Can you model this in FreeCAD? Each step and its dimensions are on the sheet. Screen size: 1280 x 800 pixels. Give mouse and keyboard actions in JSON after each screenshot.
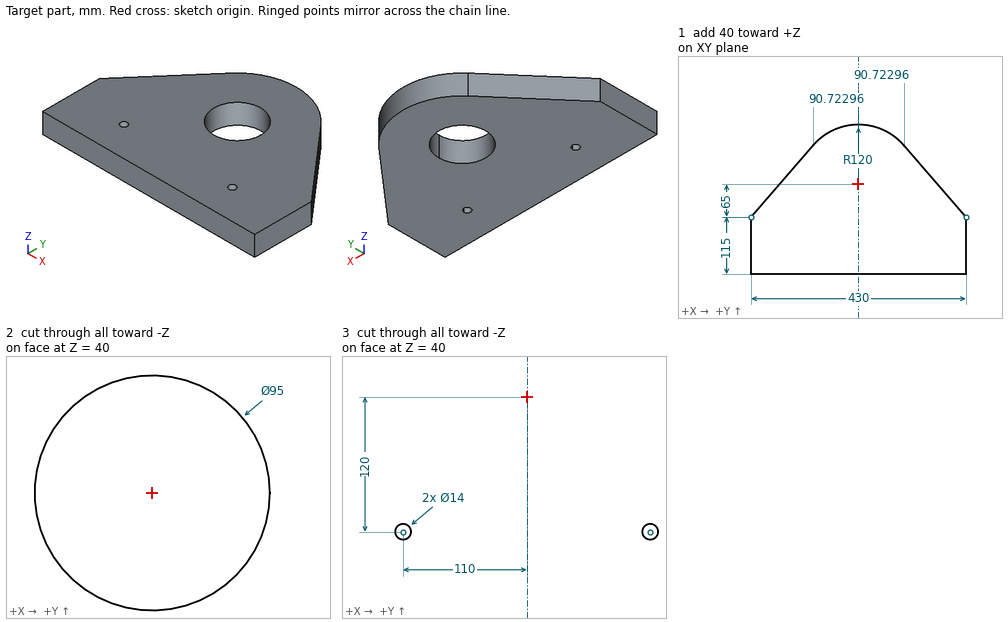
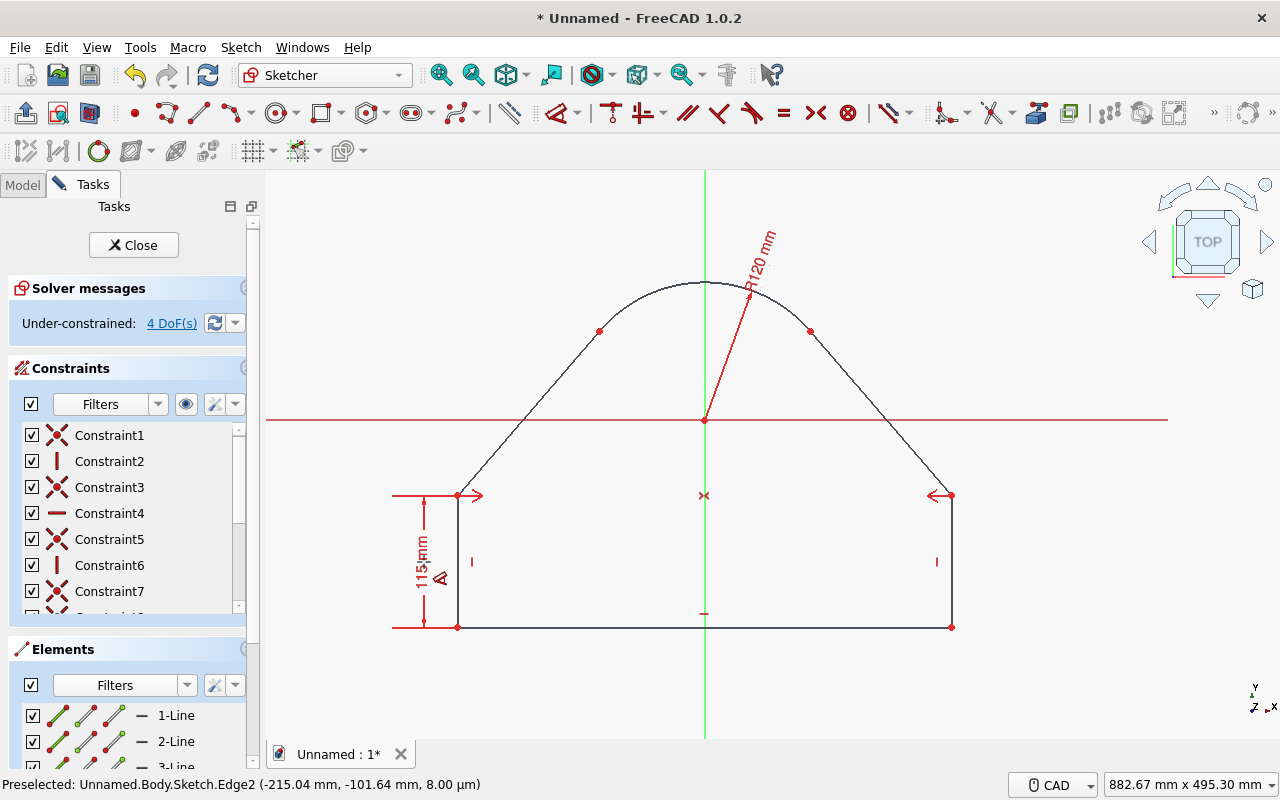
{"action": "left_click", "coordinate": [606, 628]}
{"action": "left_click", "coordinate": [591, 662]}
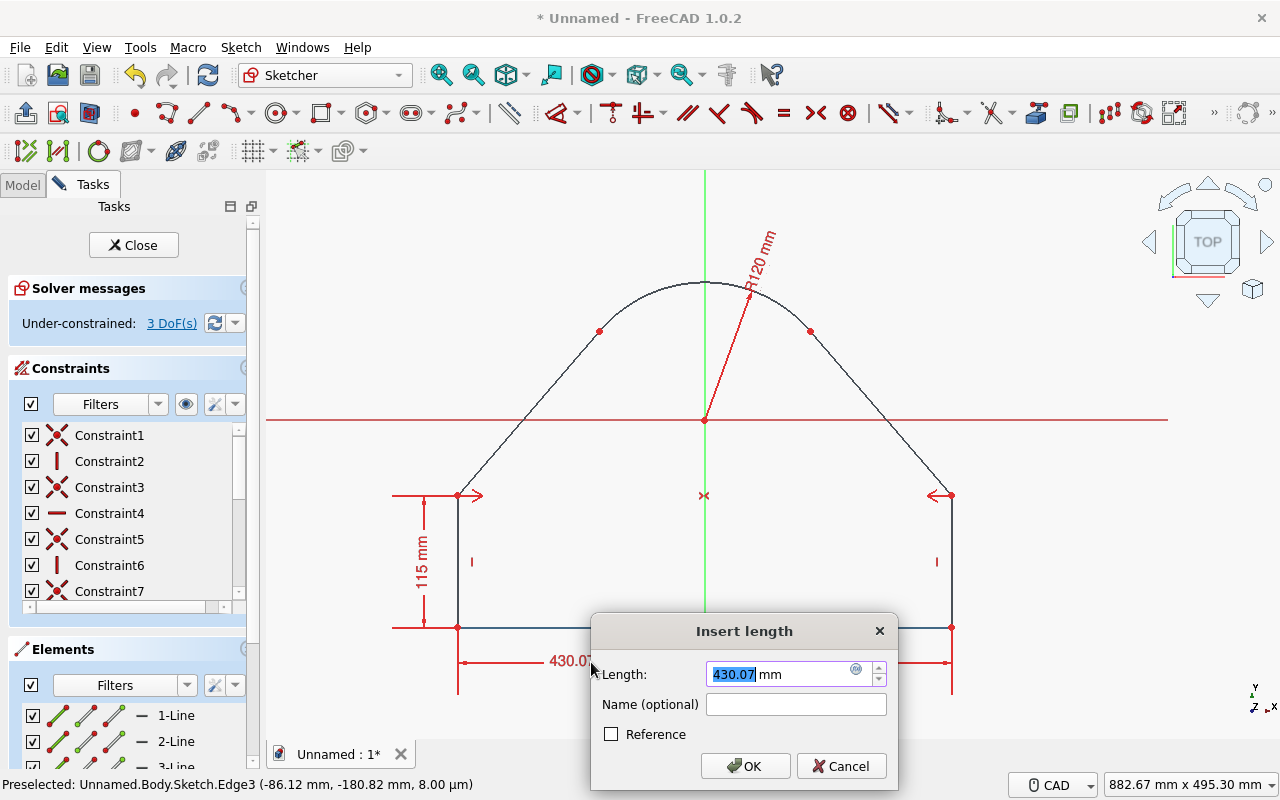
{"action": "type", "text": "430"}
{"action": "key", "text": "Return"}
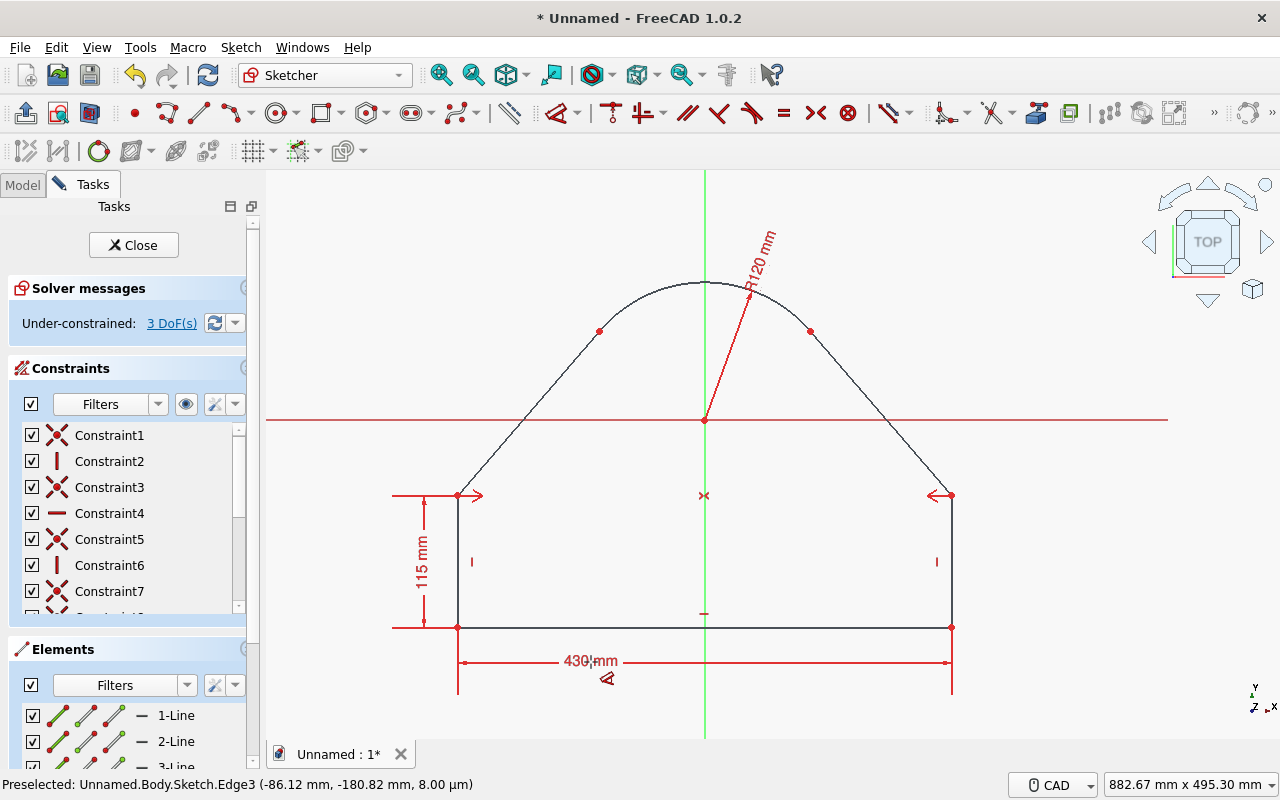
{"action": "left_click", "coordinate": [458, 496]}
{"action": "left_click", "coordinate": [424, 458]}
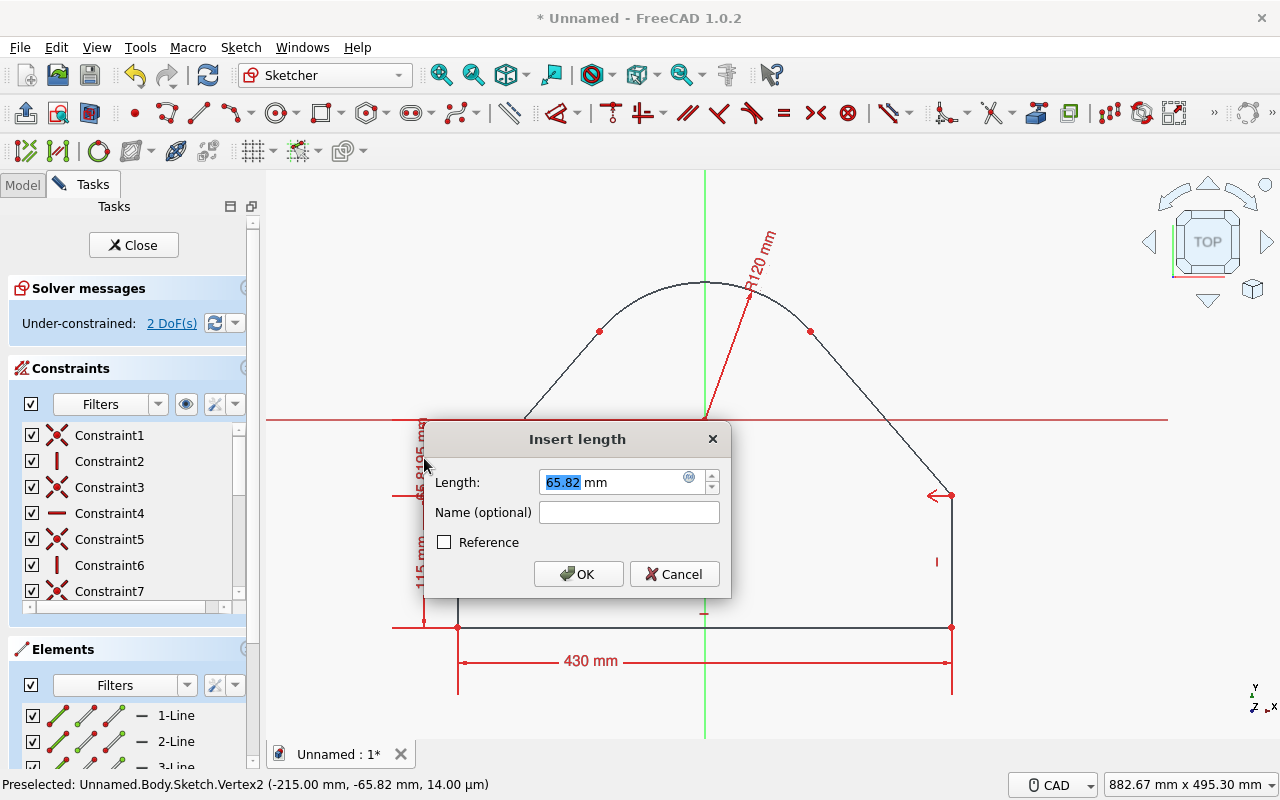
{"action": "type", "text": "65"}
{"action": "key", "text": "Return"}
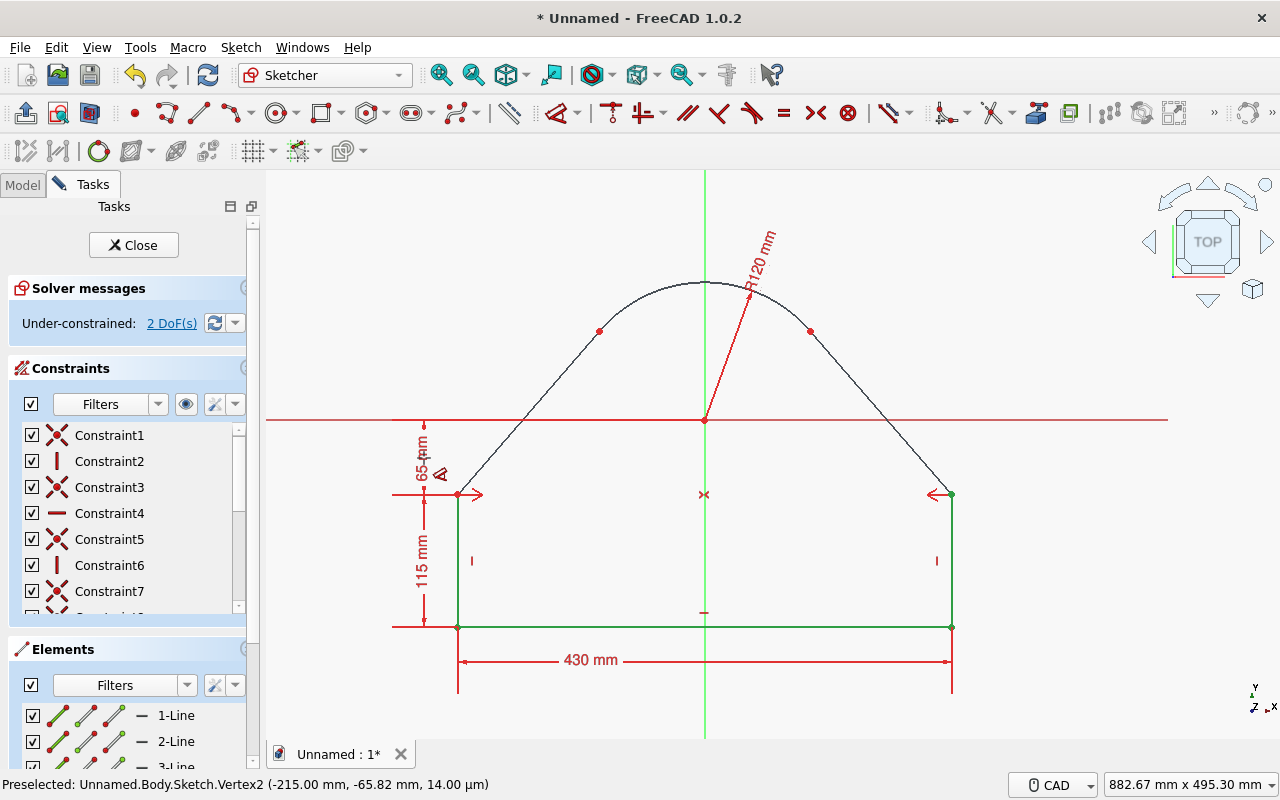
{"action": "left_click", "coordinate": [600, 331]}
{"action": "left_click", "coordinate": [615, 297]}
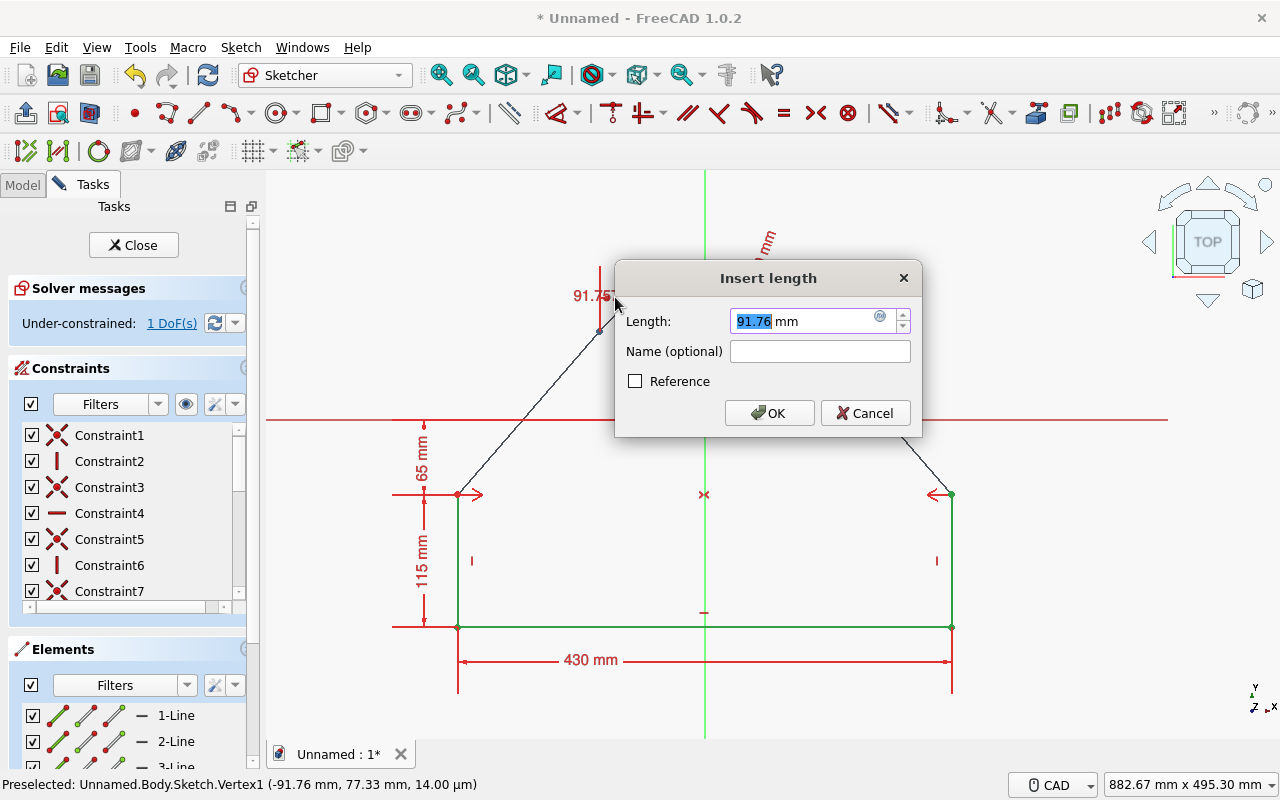
{"action": "type", "text": "90.72296"}
{"action": "key", "text": "Return"}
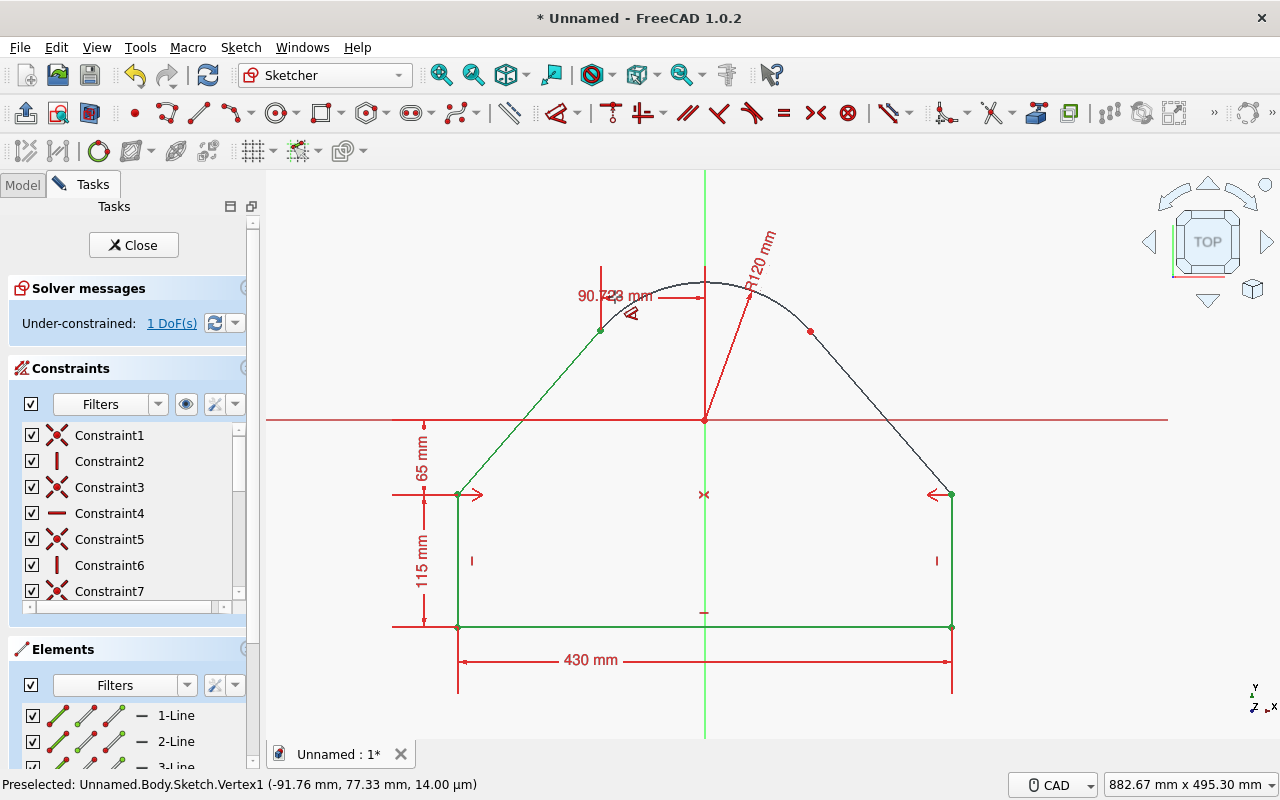
{"action": "left_click", "coordinate": [810, 331]}
{"action": "left_click", "coordinate": [721, 297]}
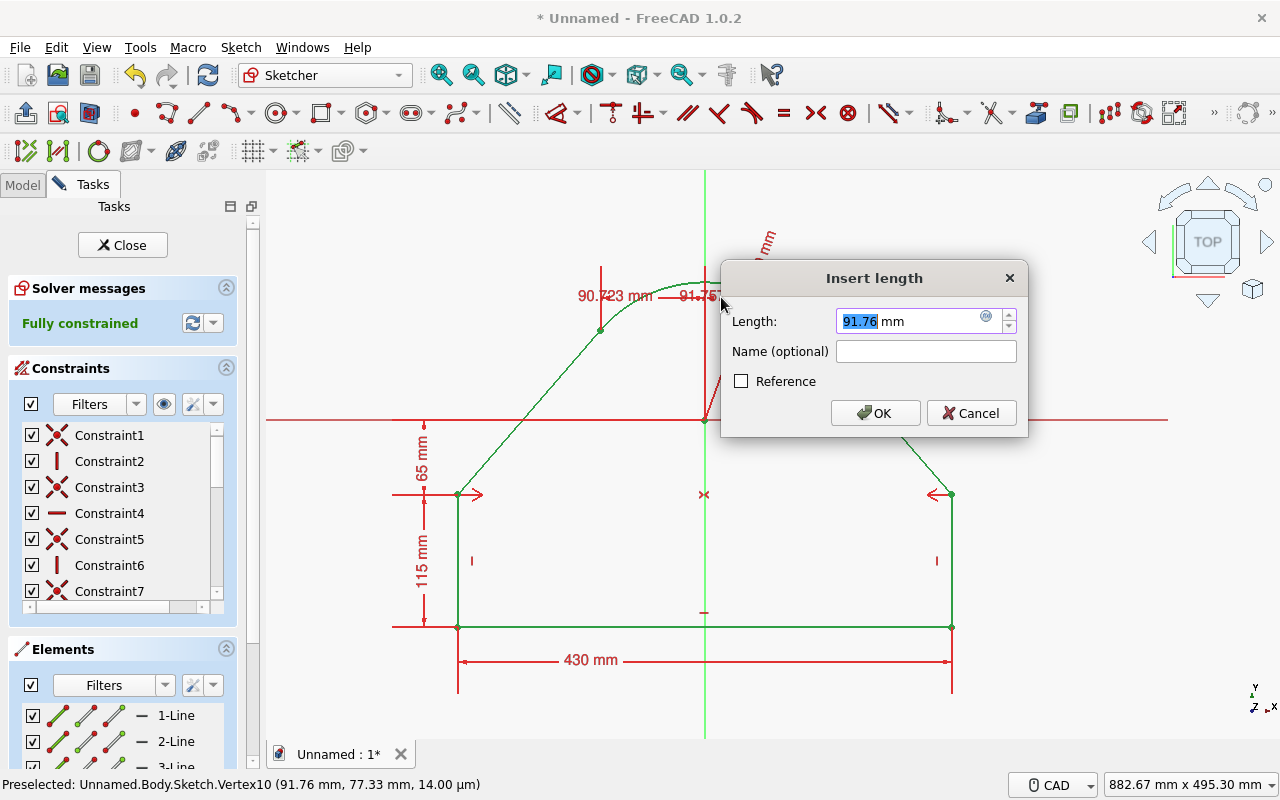
{"action": "type", "text": "90.72296"}
{"action": "key", "text": "Return"}
{"action": "key", "text": "Escape"}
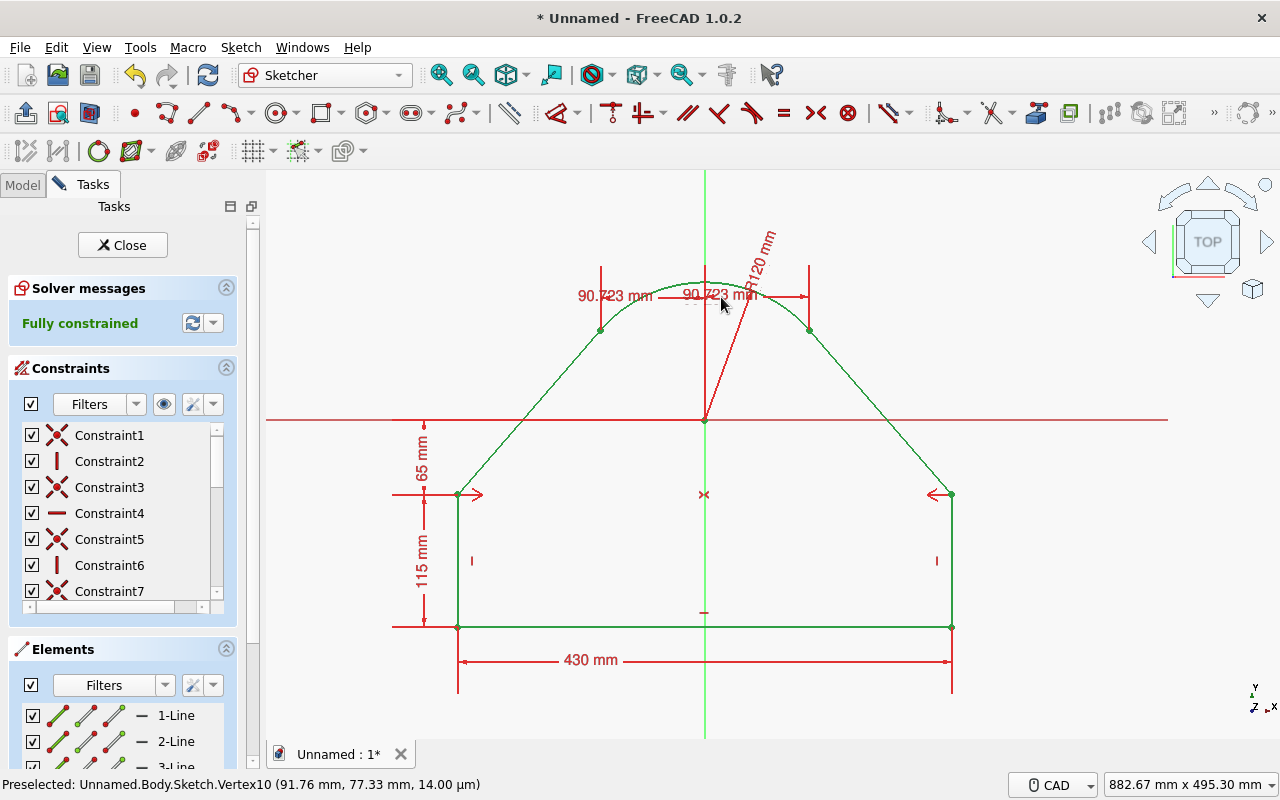
{"action": "left_click", "coordinate": [123, 245]}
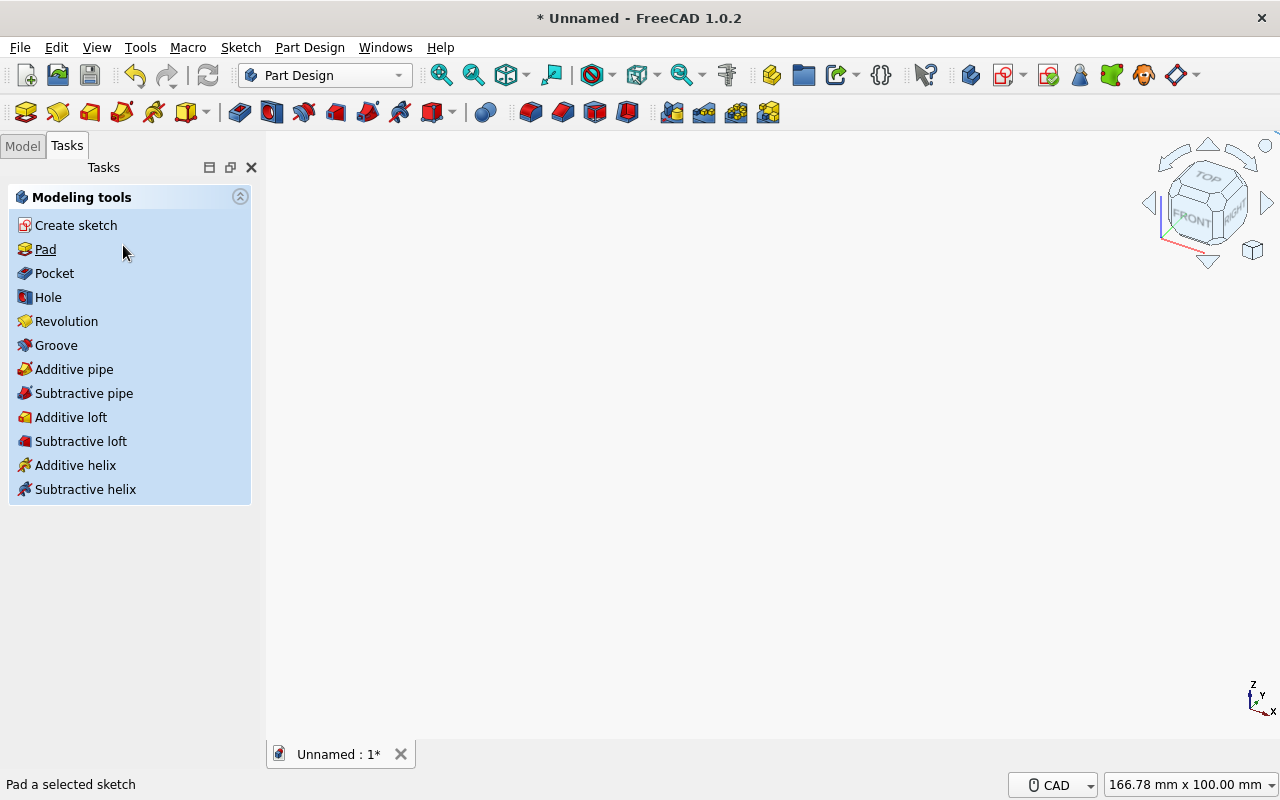
{"action": "left_click", "coordinate": [26, 112]}